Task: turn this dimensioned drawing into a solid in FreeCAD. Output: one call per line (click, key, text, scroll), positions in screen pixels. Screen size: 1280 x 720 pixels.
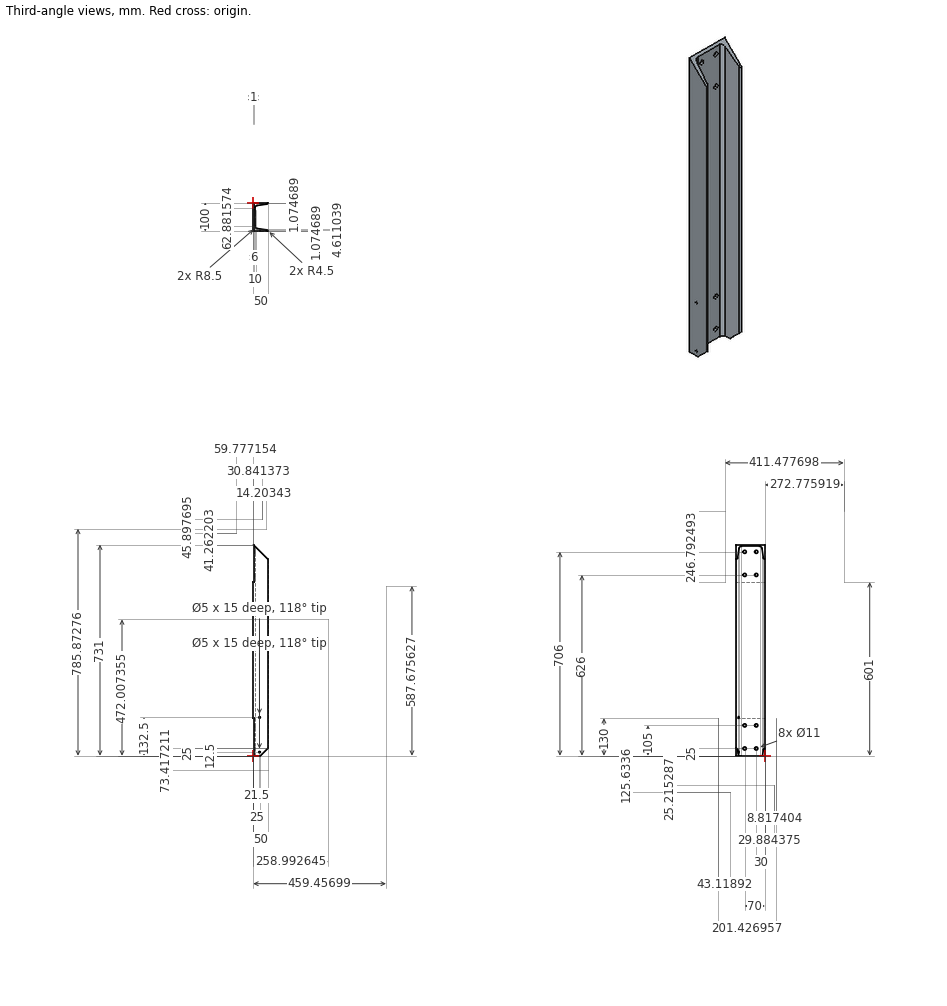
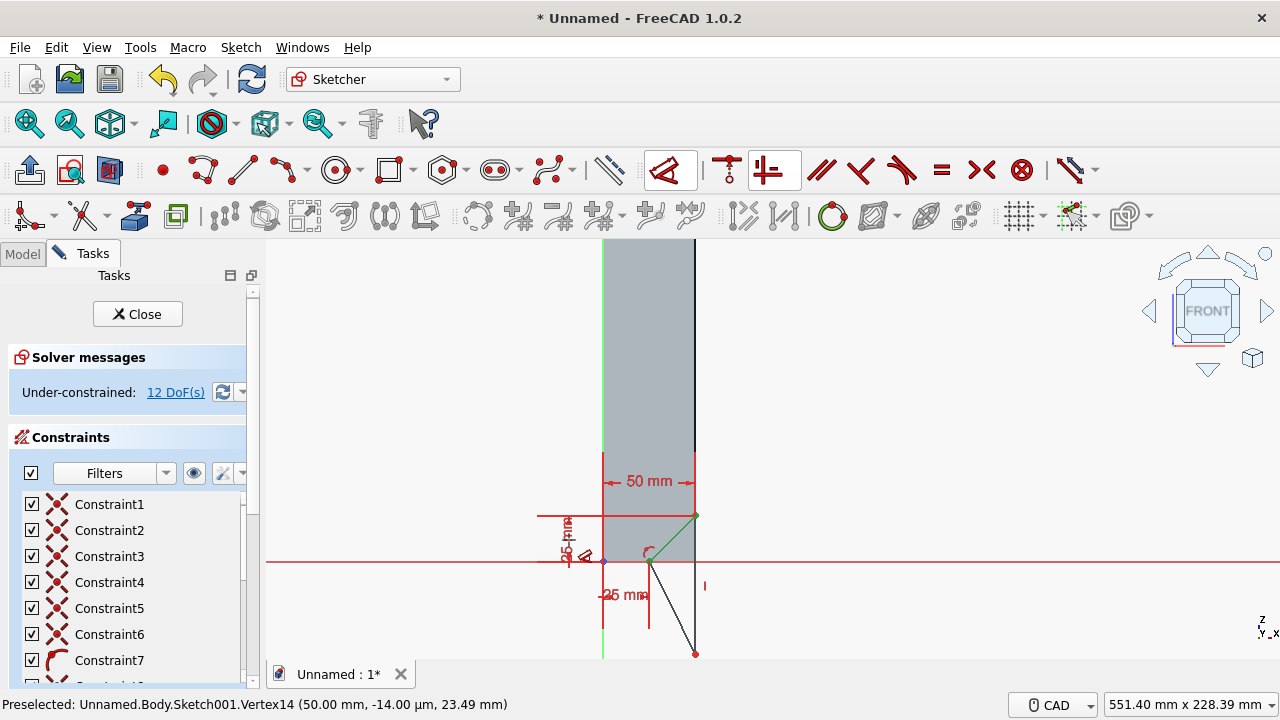
scroll(652, 567, down, 9)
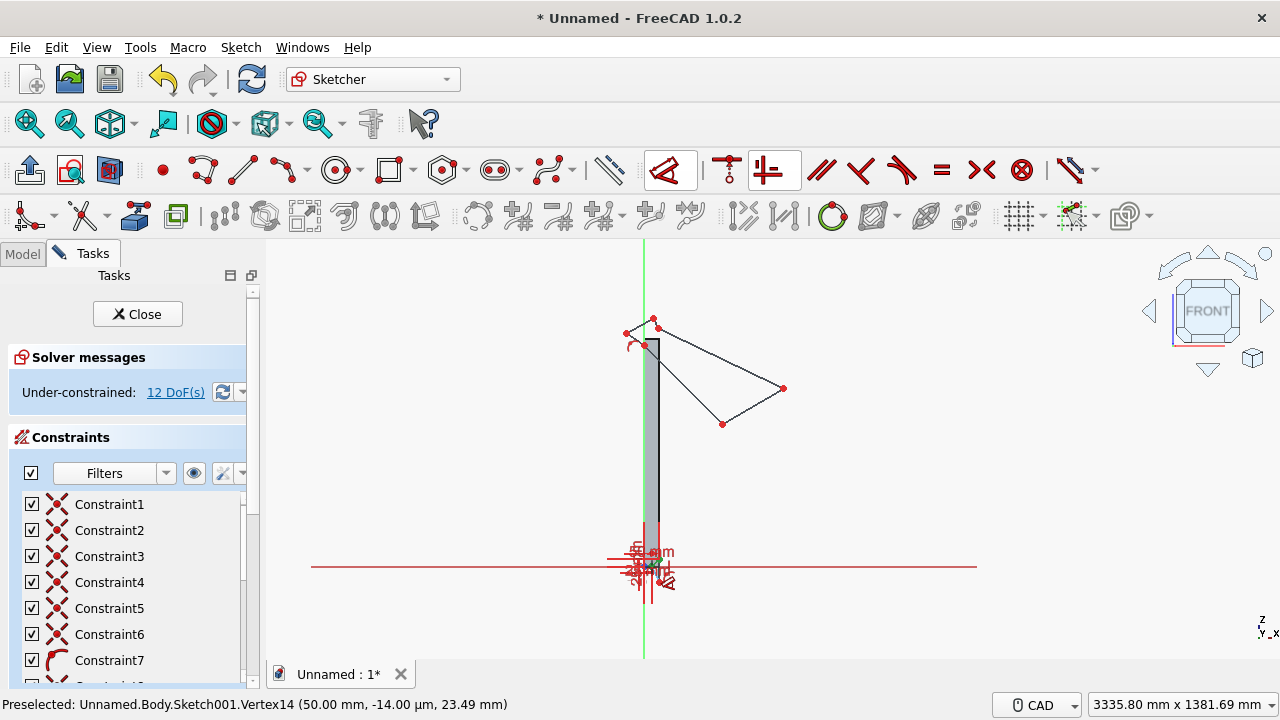
click(644, 345)
click(610, 456)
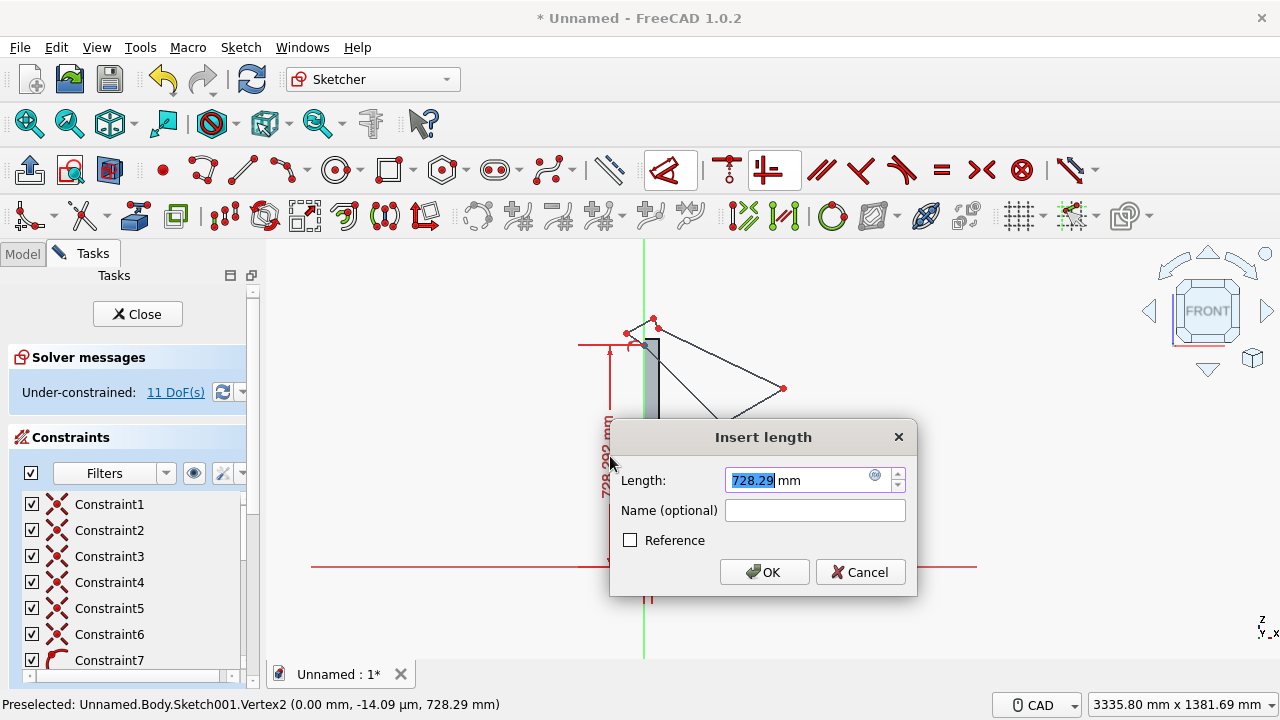
text(731)
key(Return)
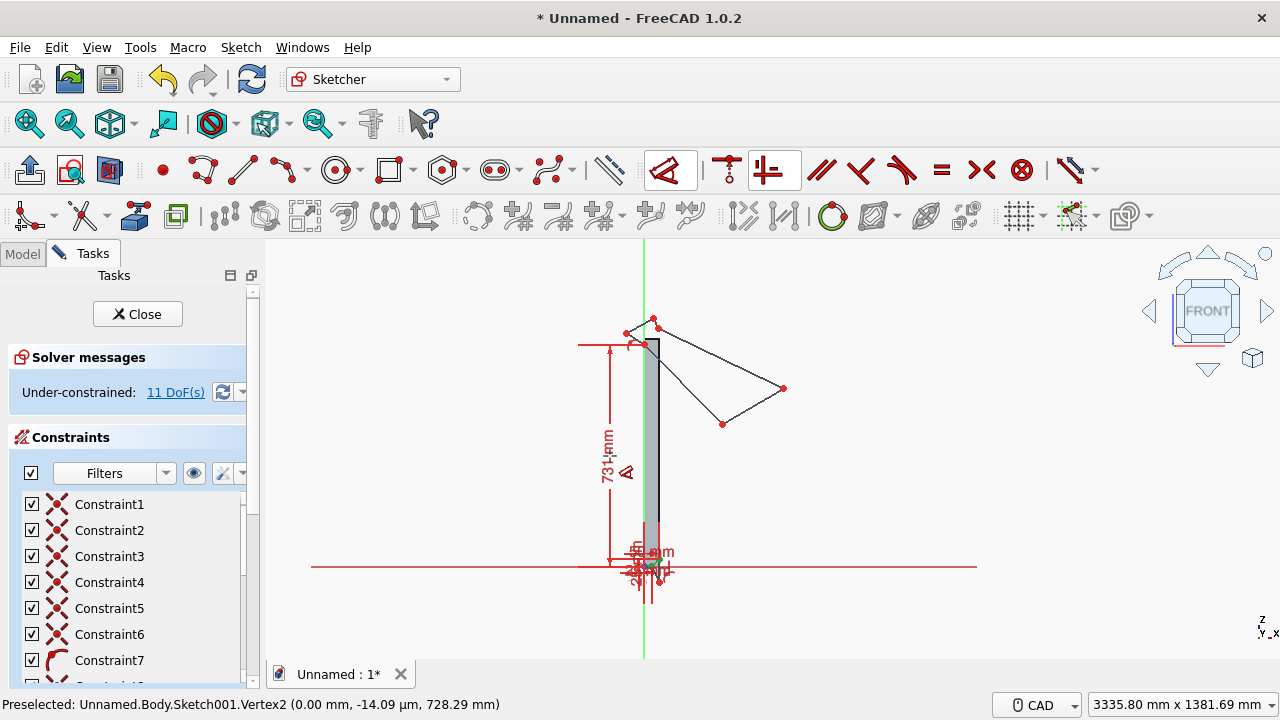
scroll(659, 568, up, 5)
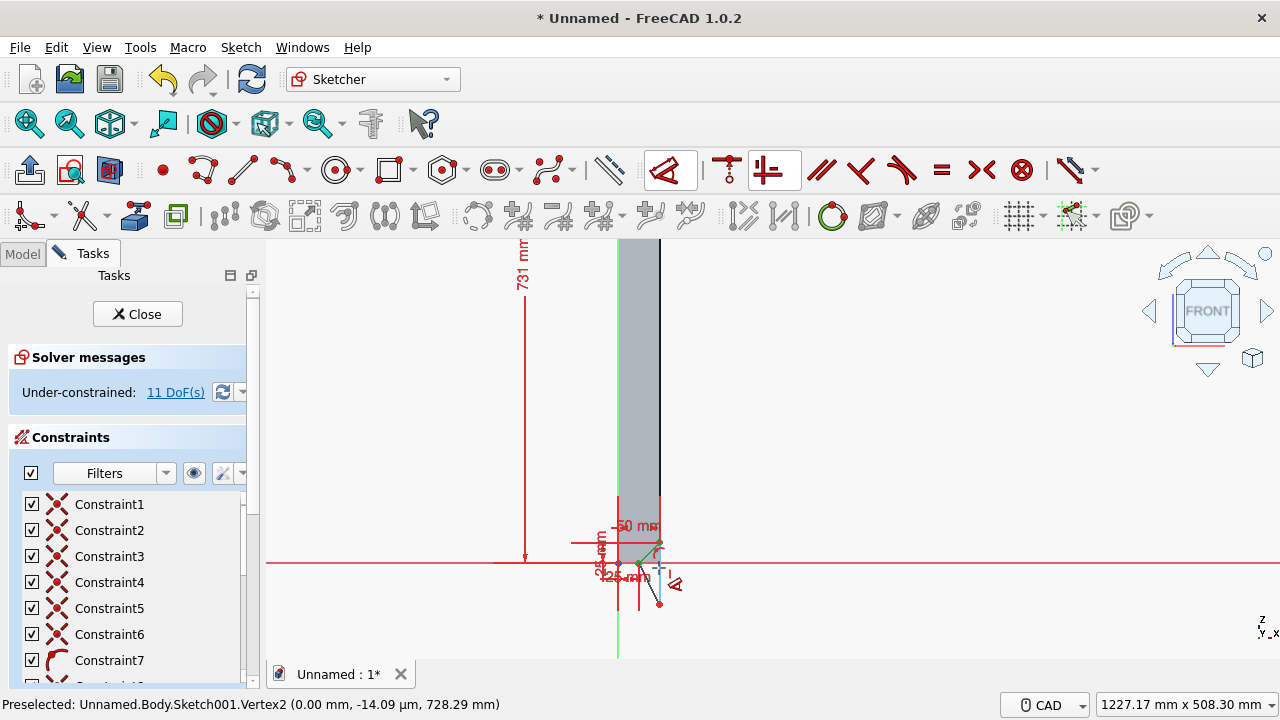
click(660, 568)
click(718, 588)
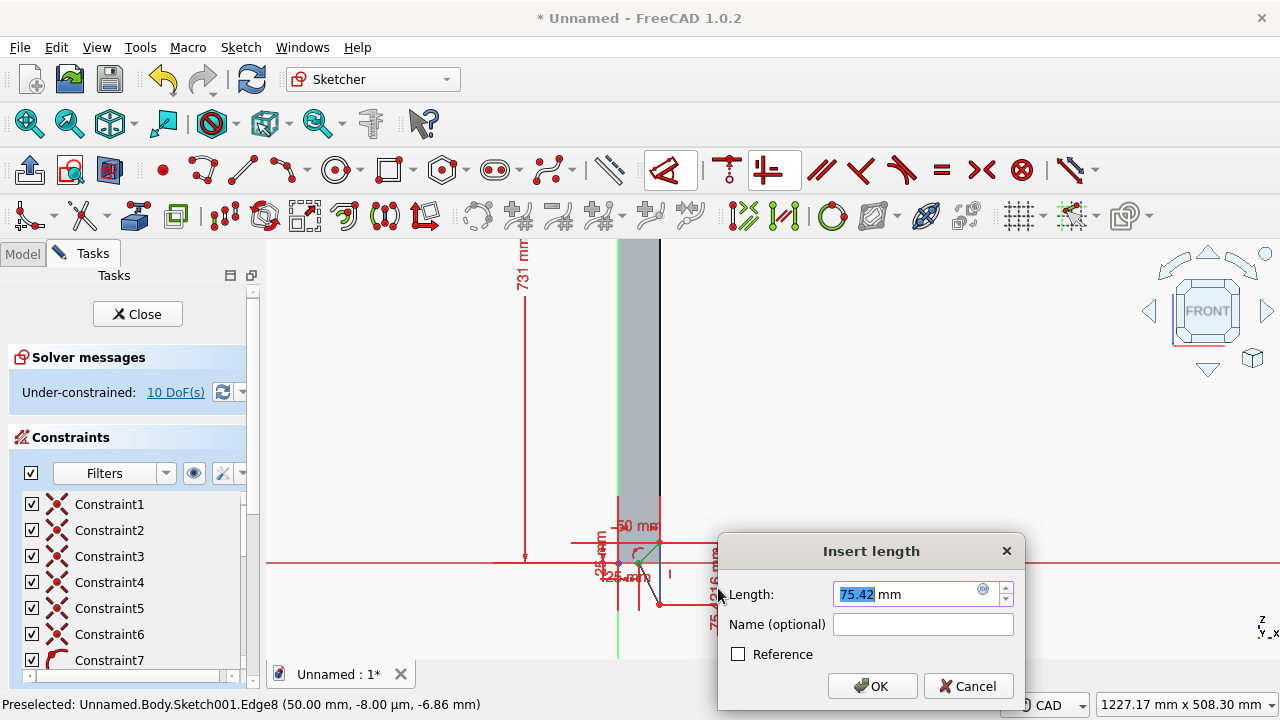
text(73.417211)
key(Return)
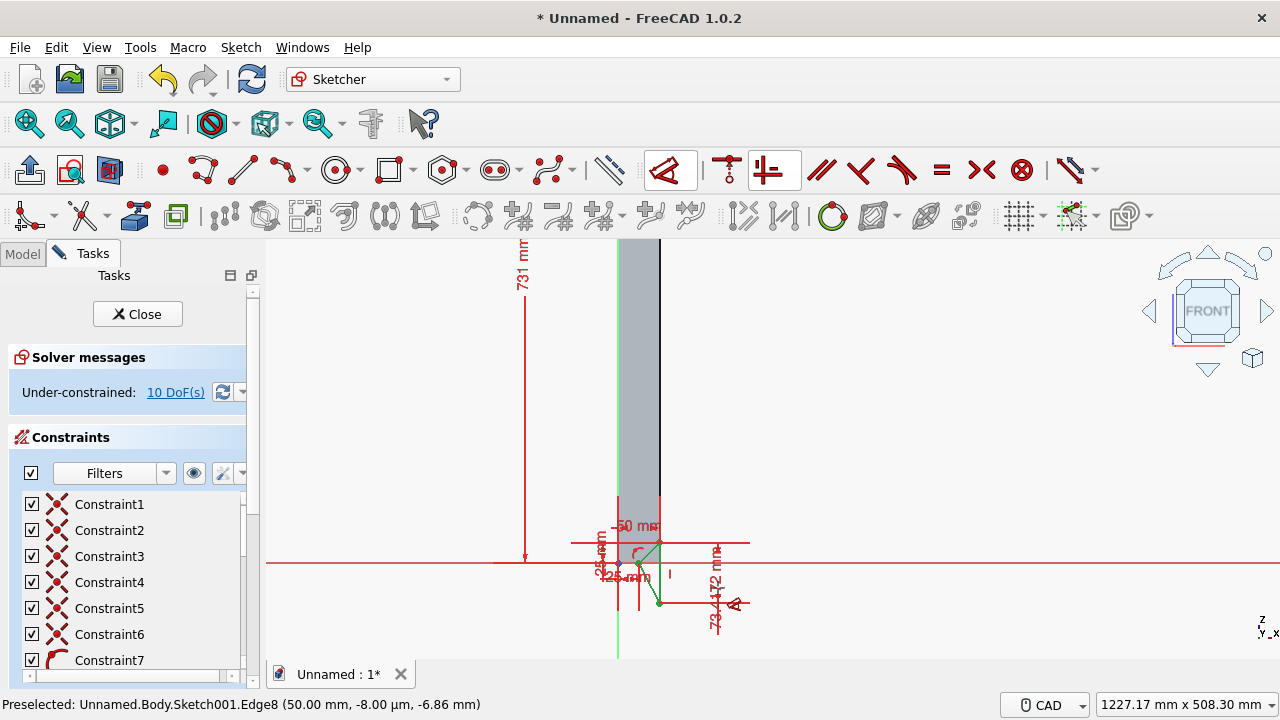
scroll(659, 568, down, 5)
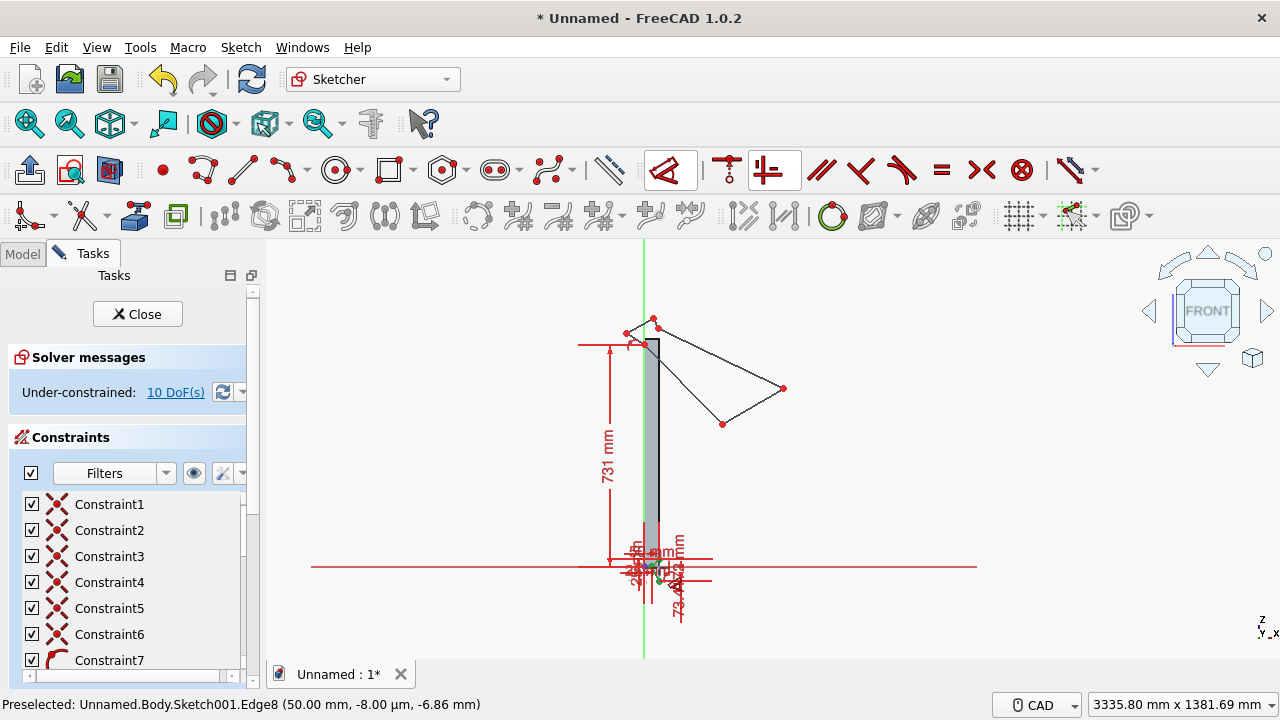
scroll(656, 322, up, 12)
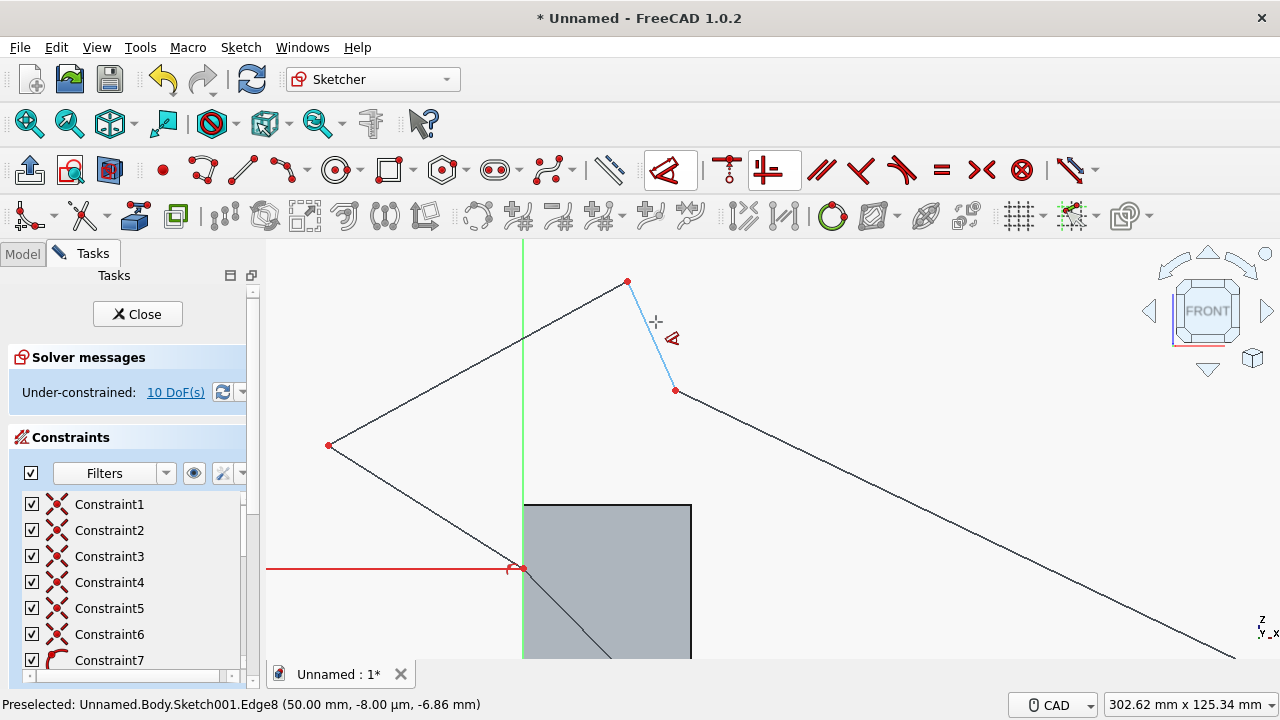
click(647, 325)
click(652, 424)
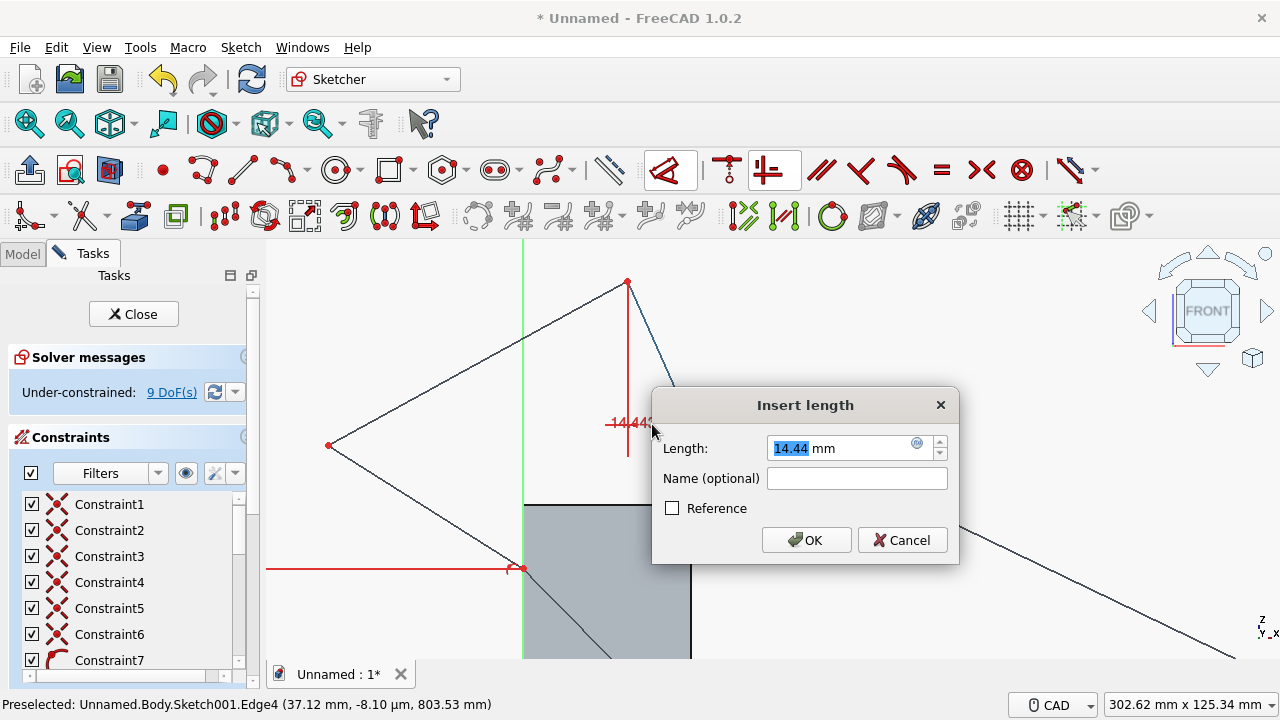
text(14.20343)
key(Return)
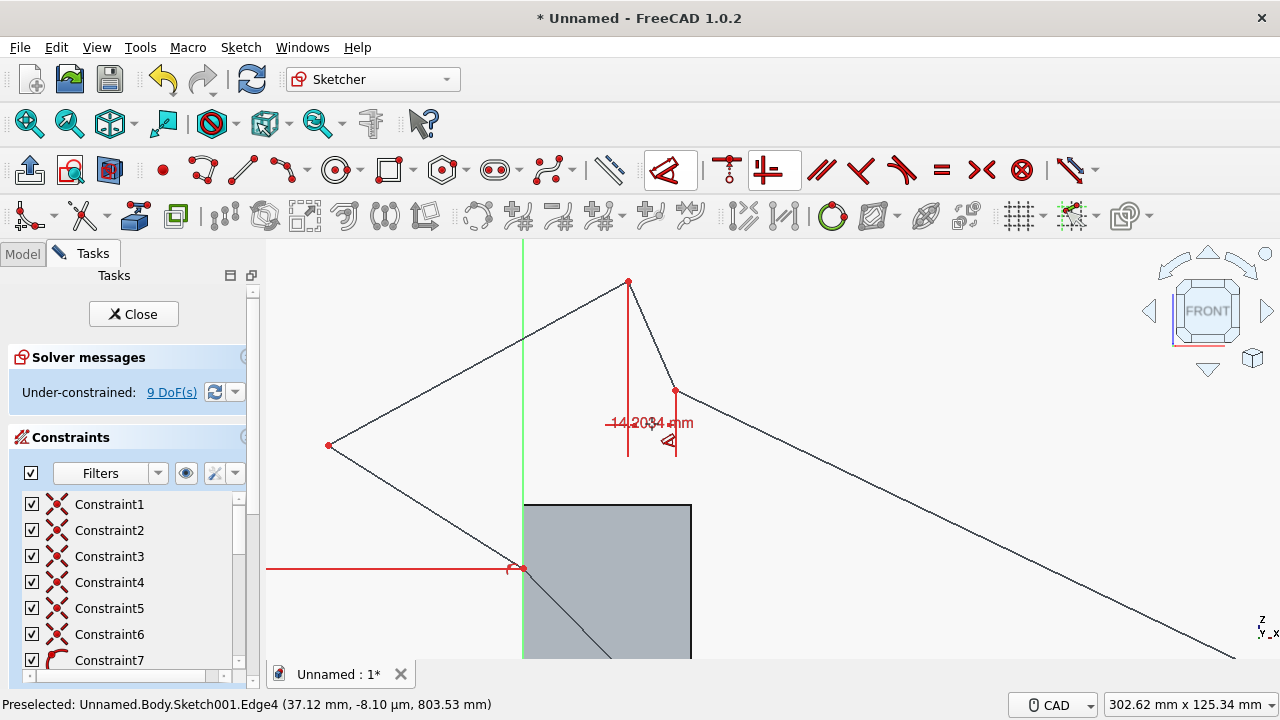
scroll(656, 321, down, 12)